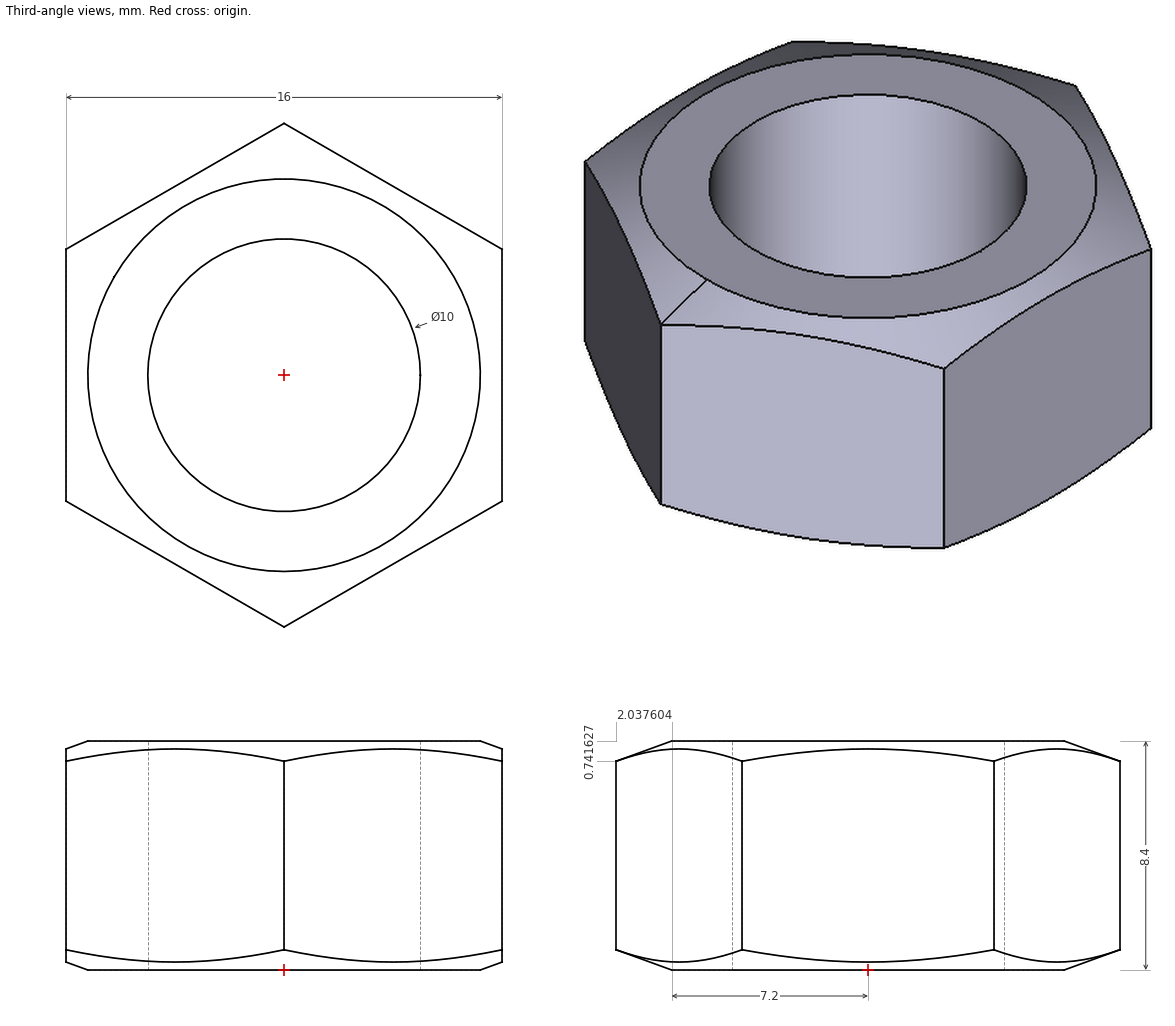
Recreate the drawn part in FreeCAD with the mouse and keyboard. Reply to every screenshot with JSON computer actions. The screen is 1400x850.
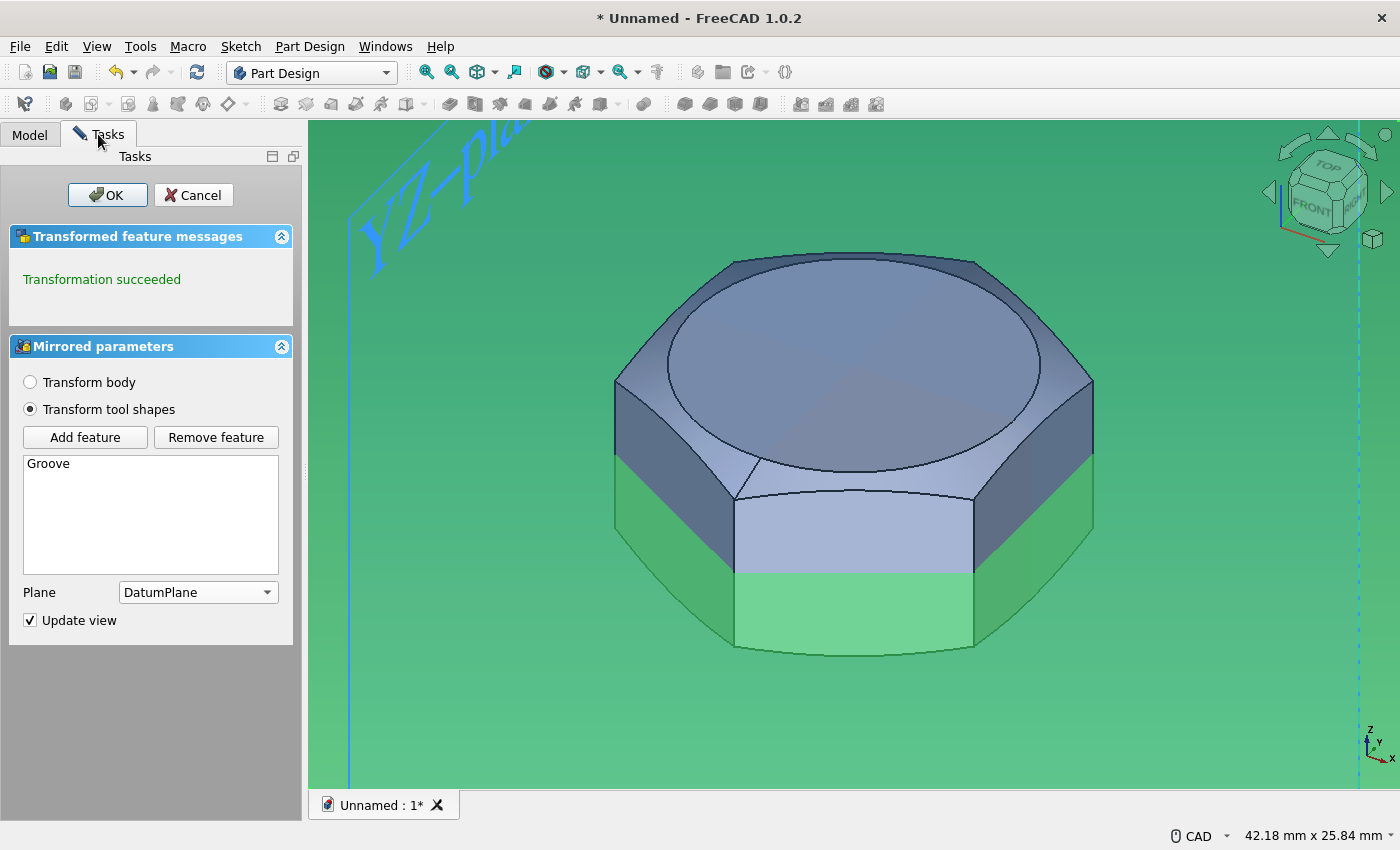
{"action": "left_click", "coordinate": [108, 195]}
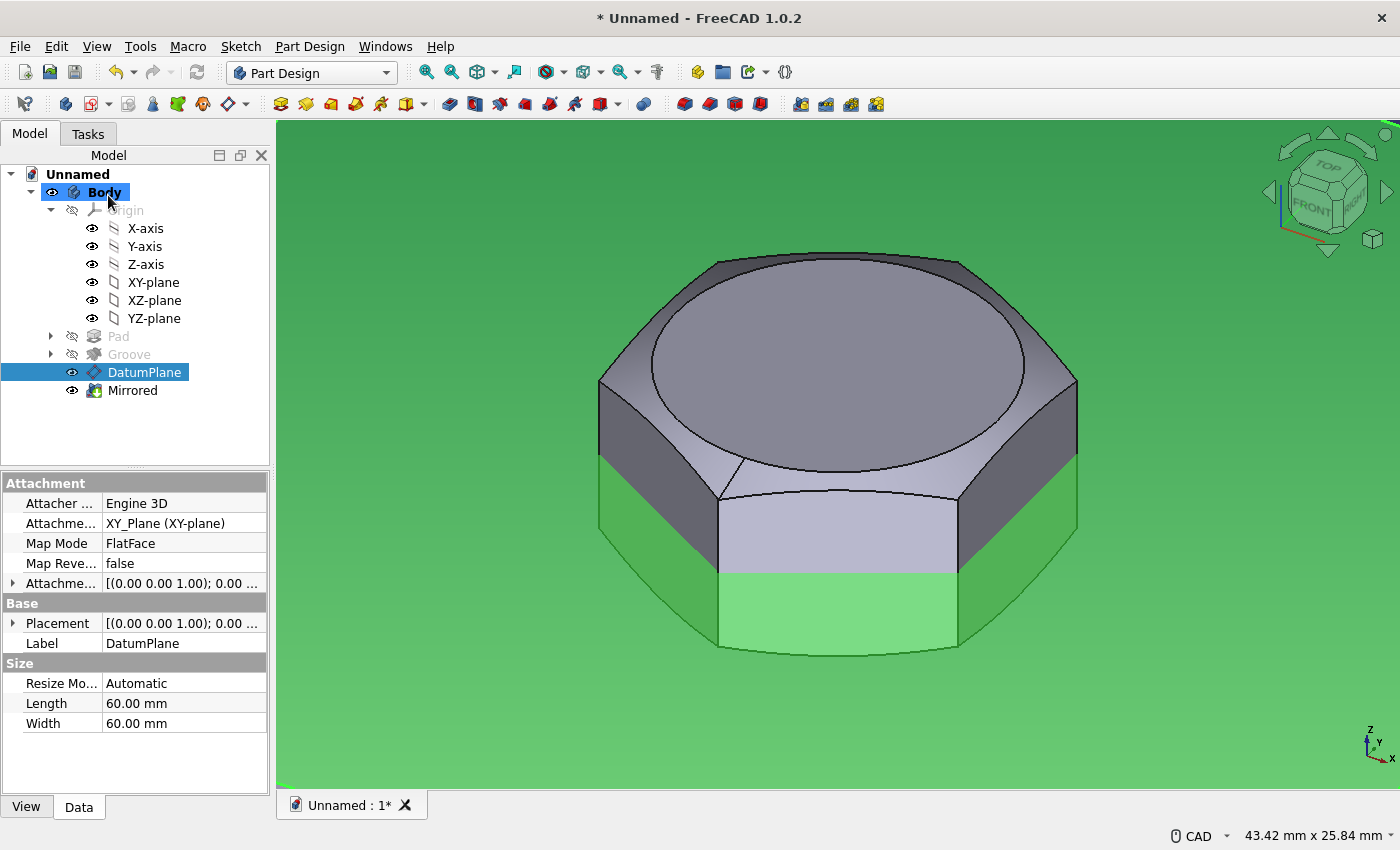
{"action": "left_click", "coordinate": [117, 372]}
{"action": "key", "text": "space"}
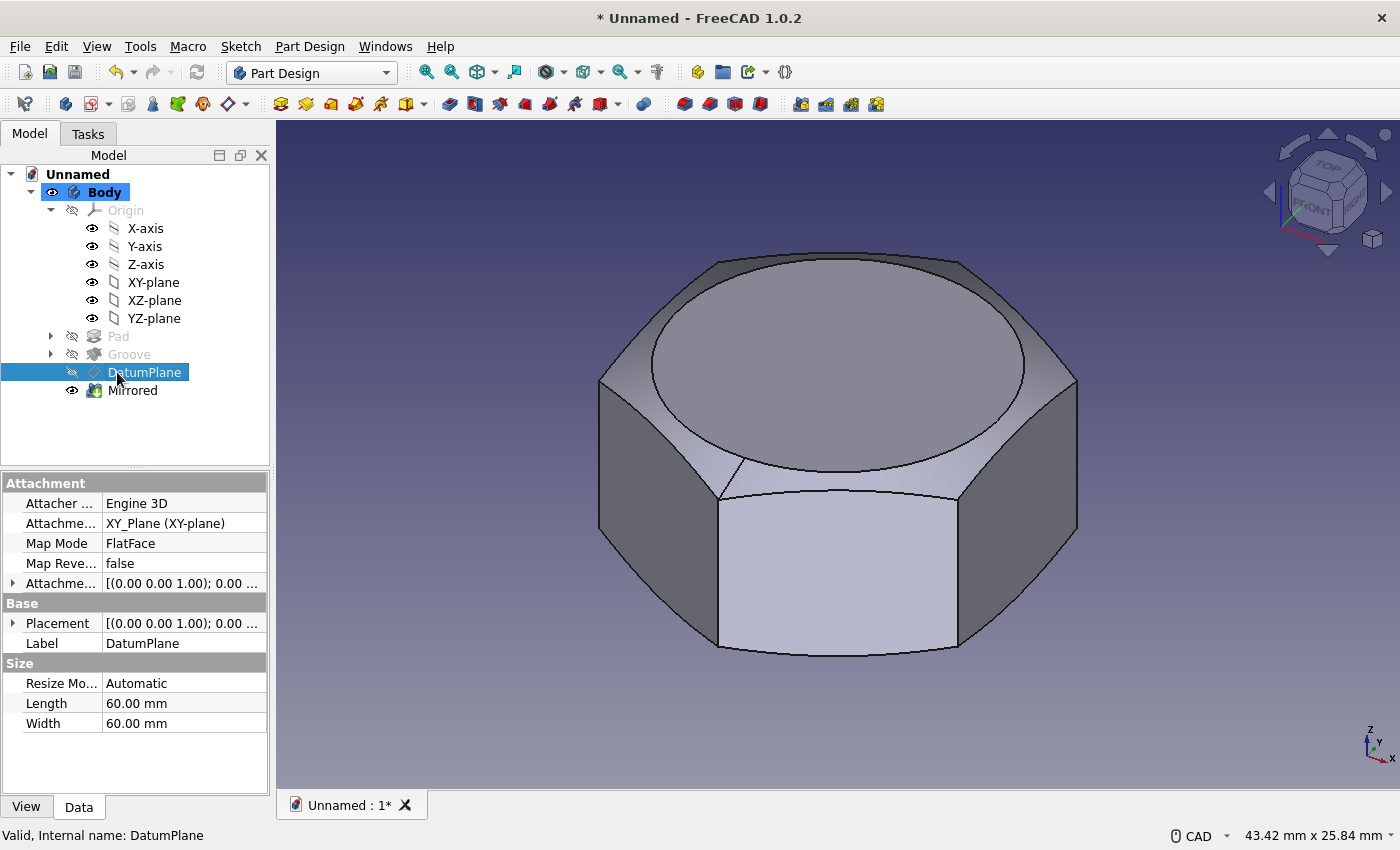
{"action": "left_click", "coordinate": [838, 364]}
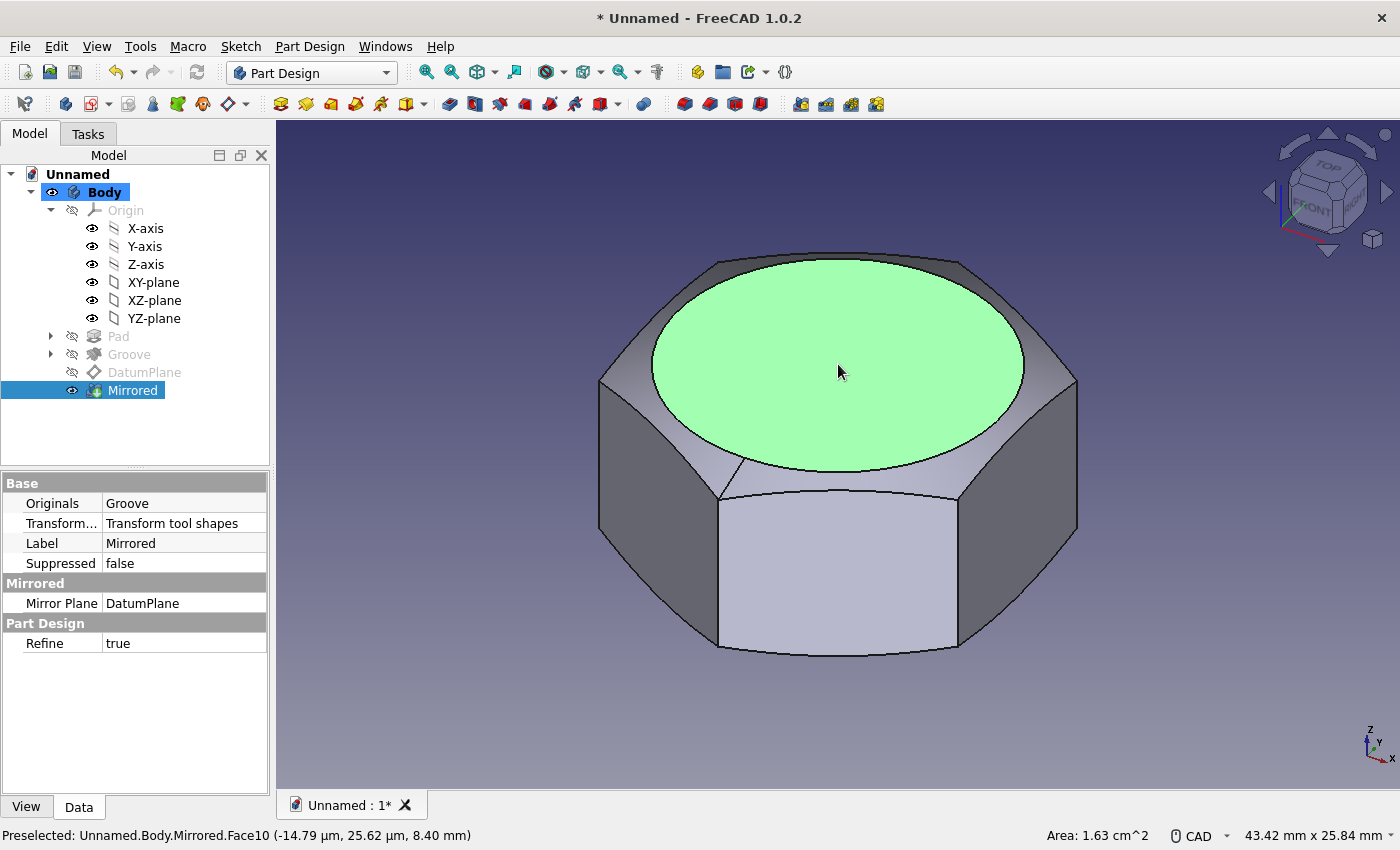
{"action": "left_click", "coordinate": [90, 104]}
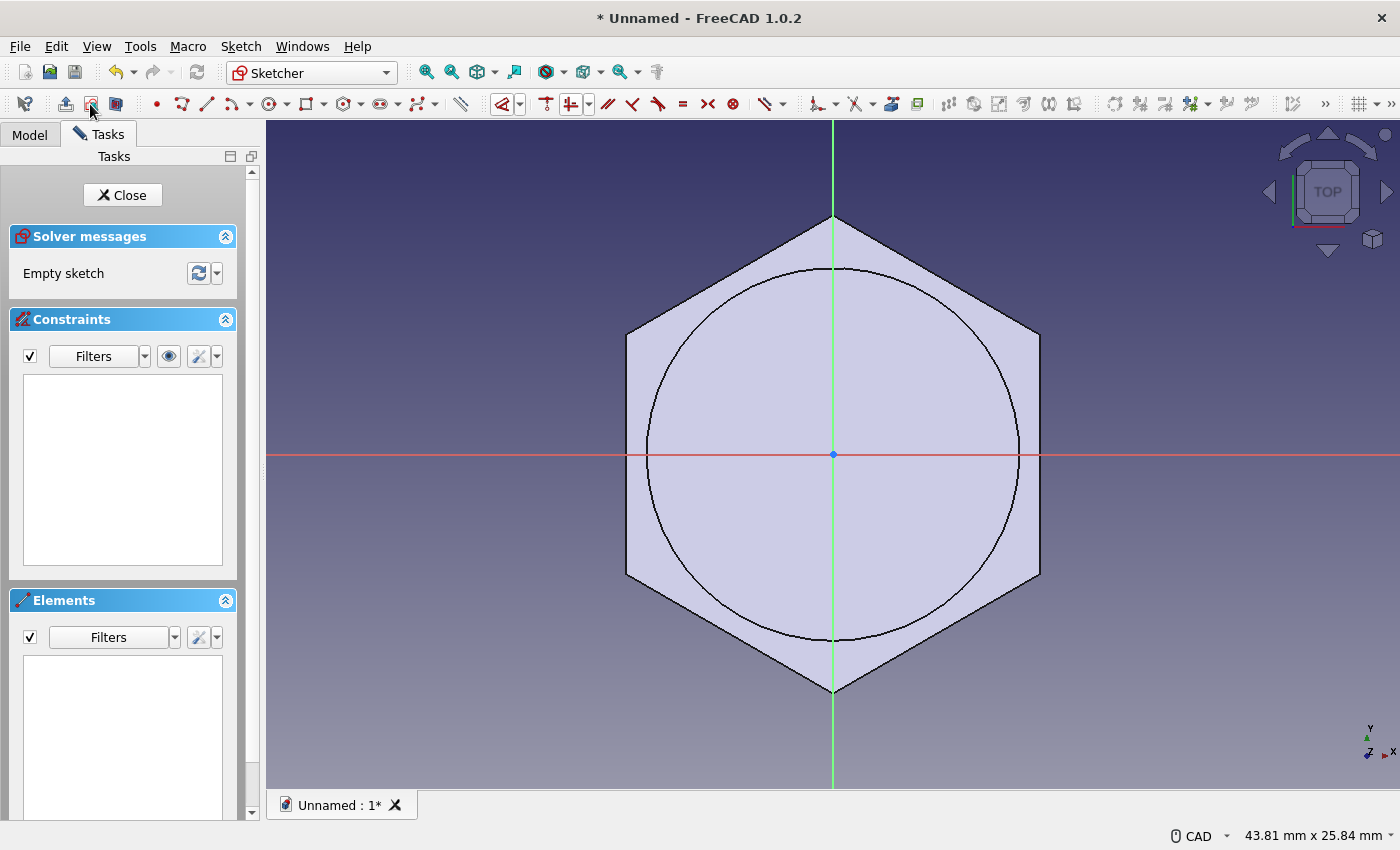
{"action": "scroll", "coordinate": [916, 454], "scroll_direction": "up", "scroll_amount": 3}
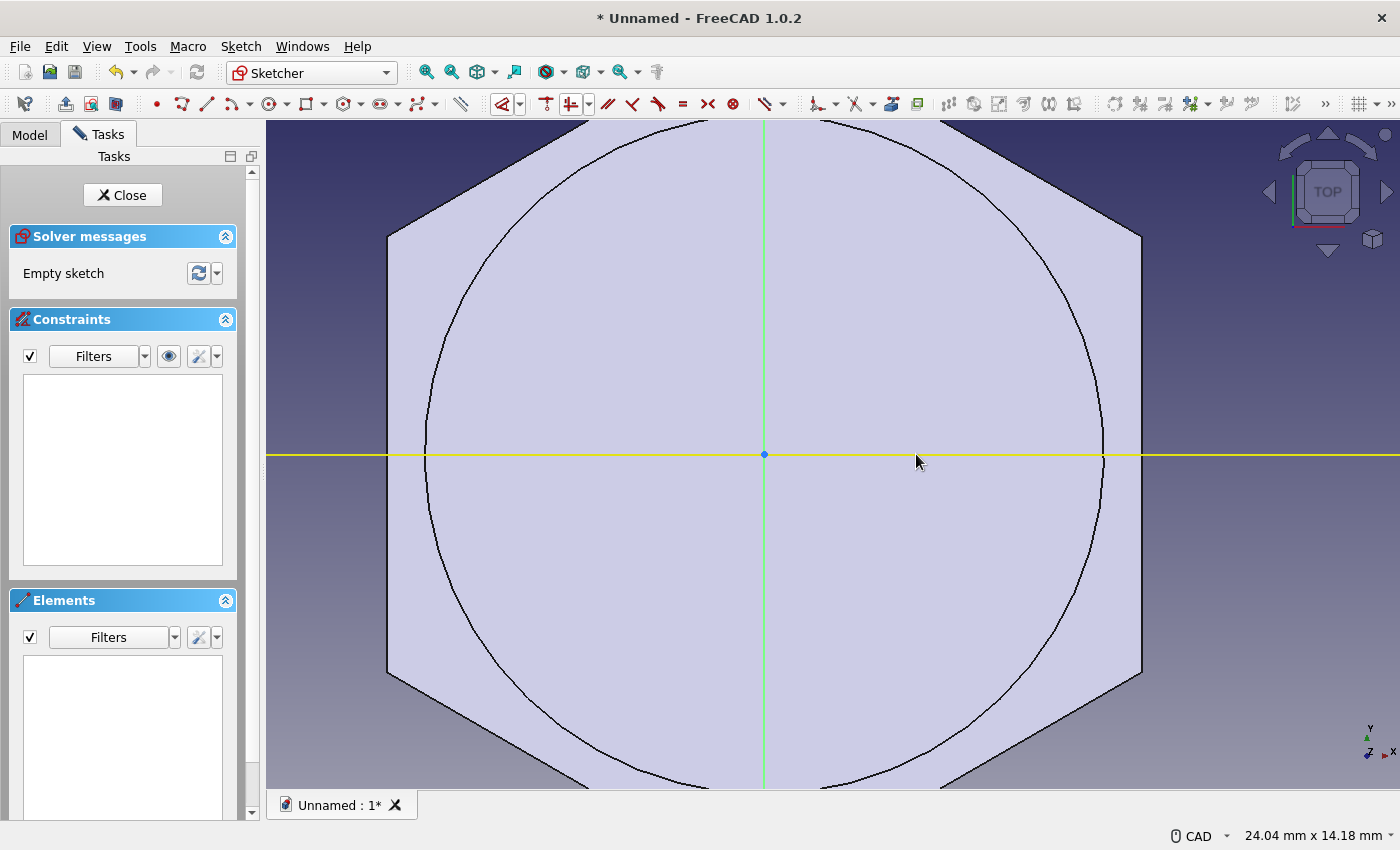
{"action": "left_click", "coordinate": [268, 104]}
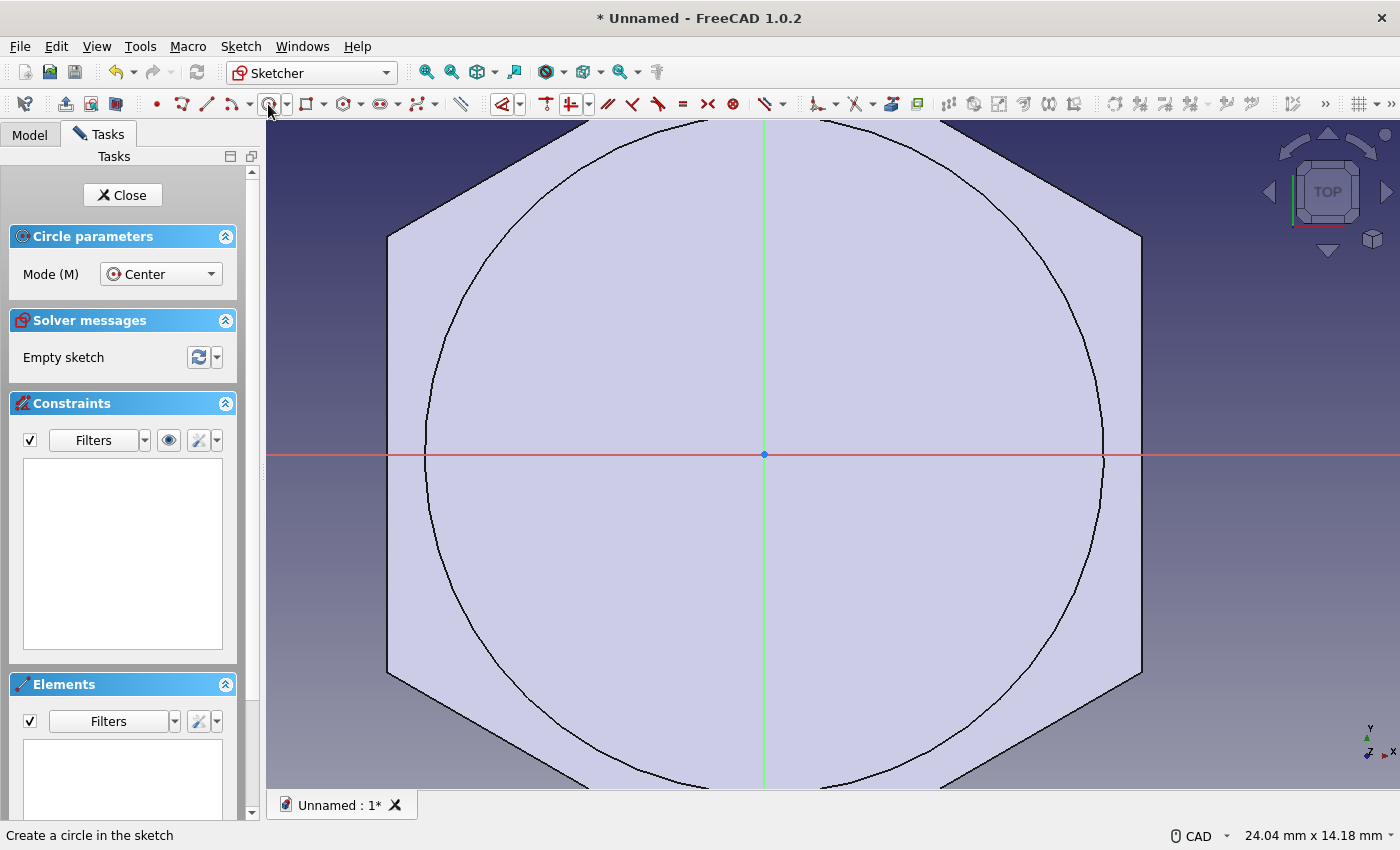
{"action": "left_click", "coordinate": [764, 454]}
{"action": "mouse_move", "coordinate": [931, 288]}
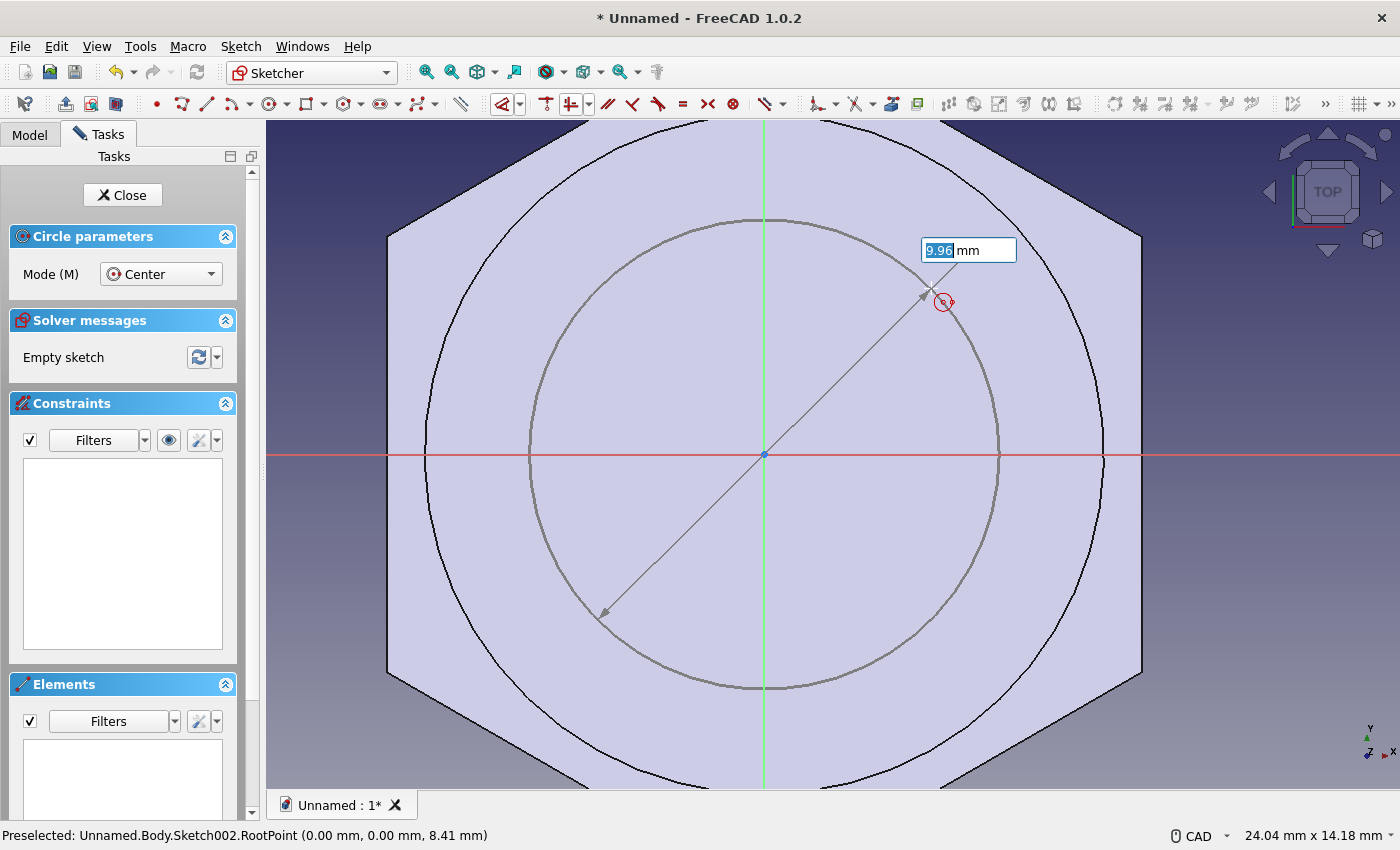
{"action": "type", "text": "10"}
{"action": "key", "text": "Return"}
{"action": "key", "text": "Escape"}